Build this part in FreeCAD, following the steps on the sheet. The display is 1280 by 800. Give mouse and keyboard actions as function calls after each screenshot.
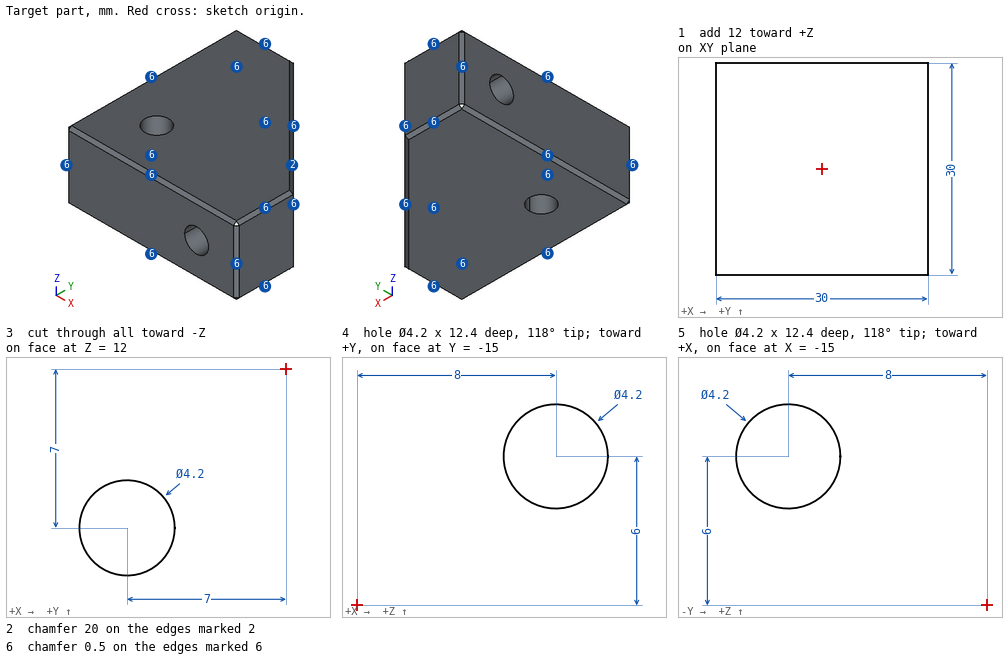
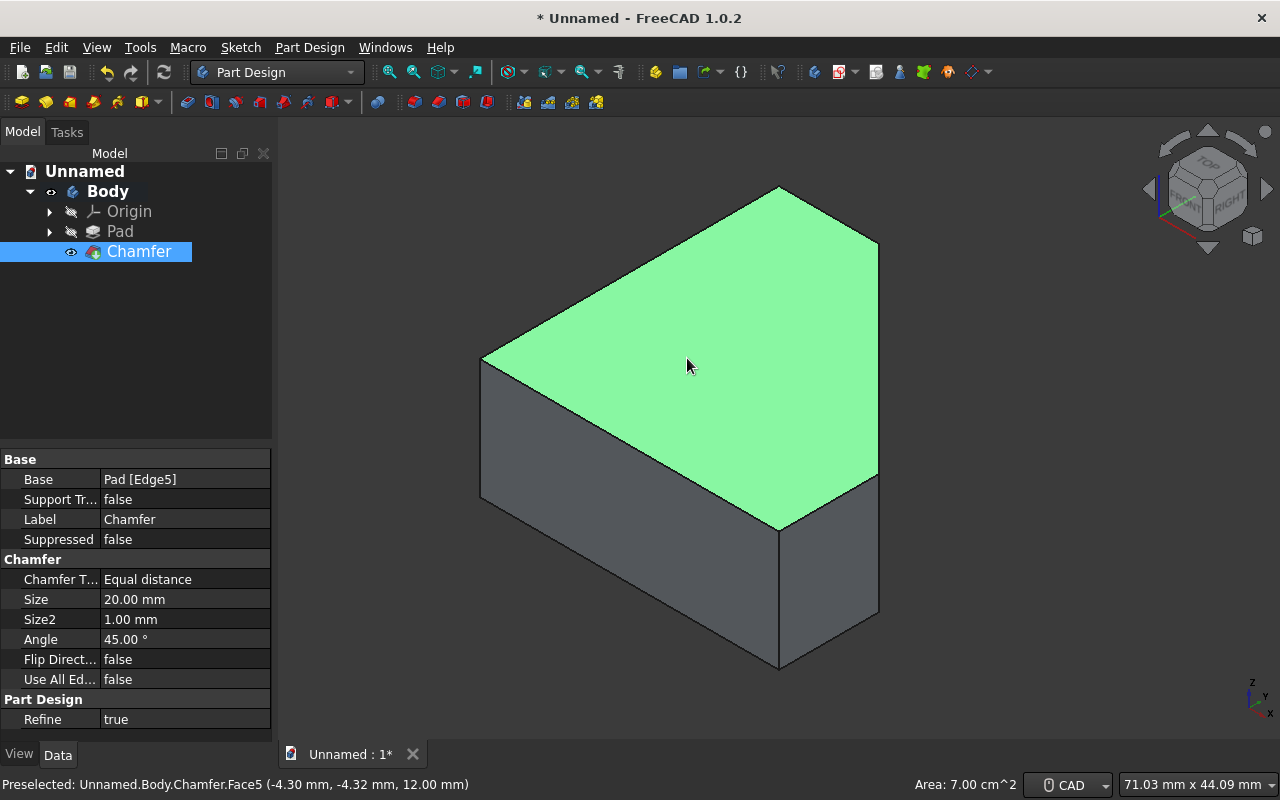
click(840, 72)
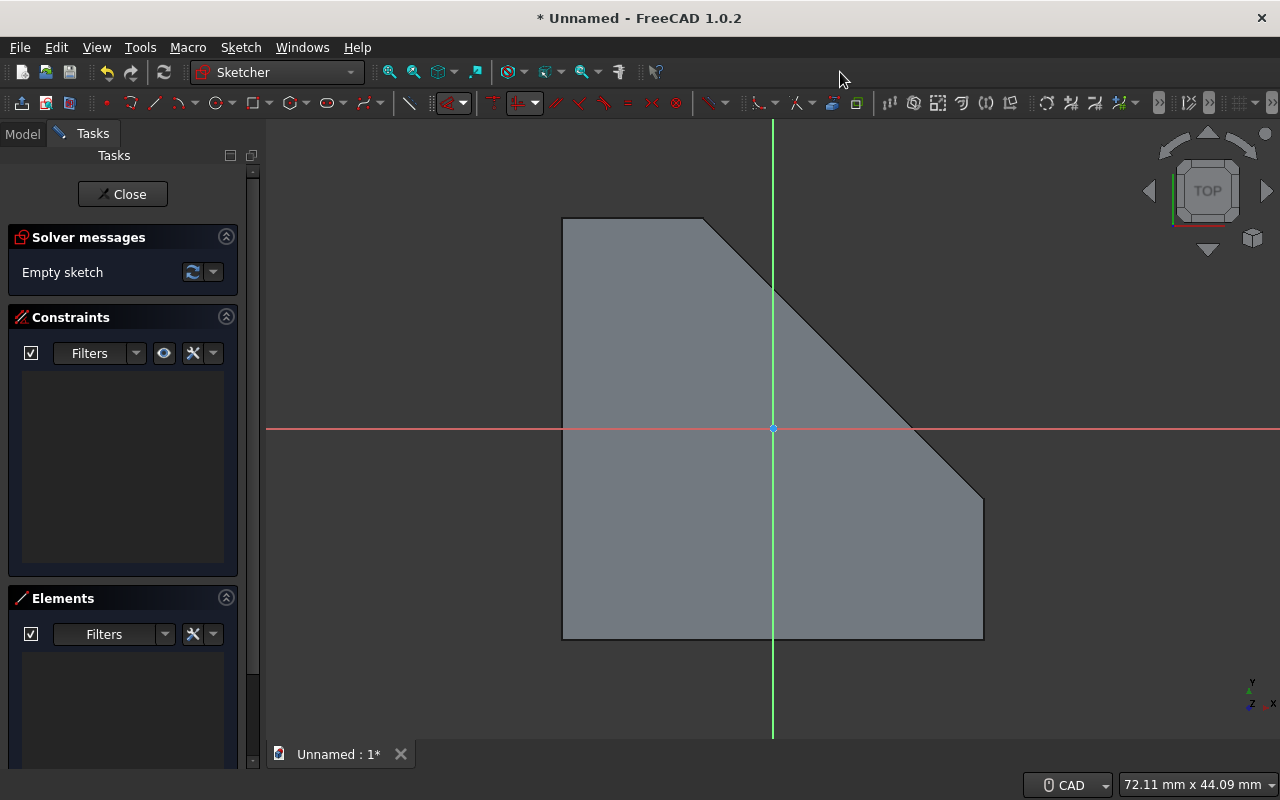
scroll(711, 521, up, 6)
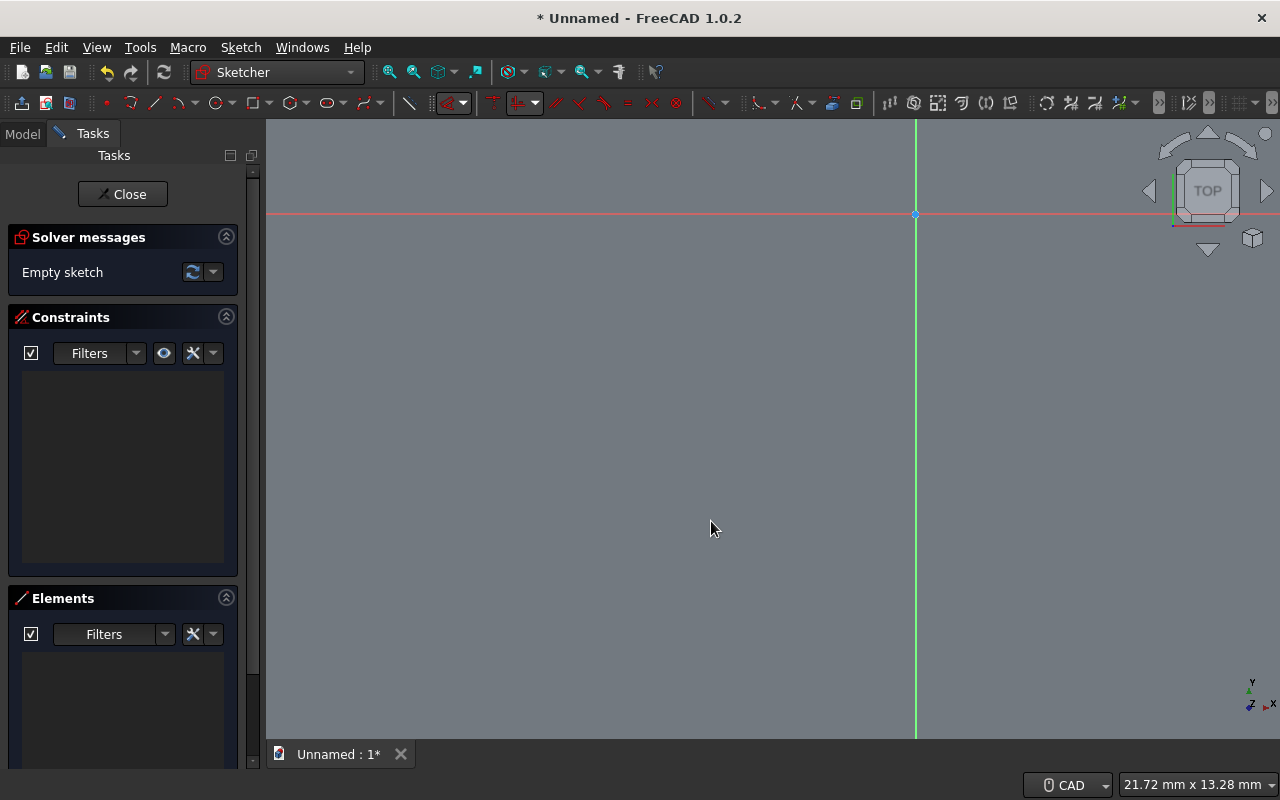
key(g)
key(c)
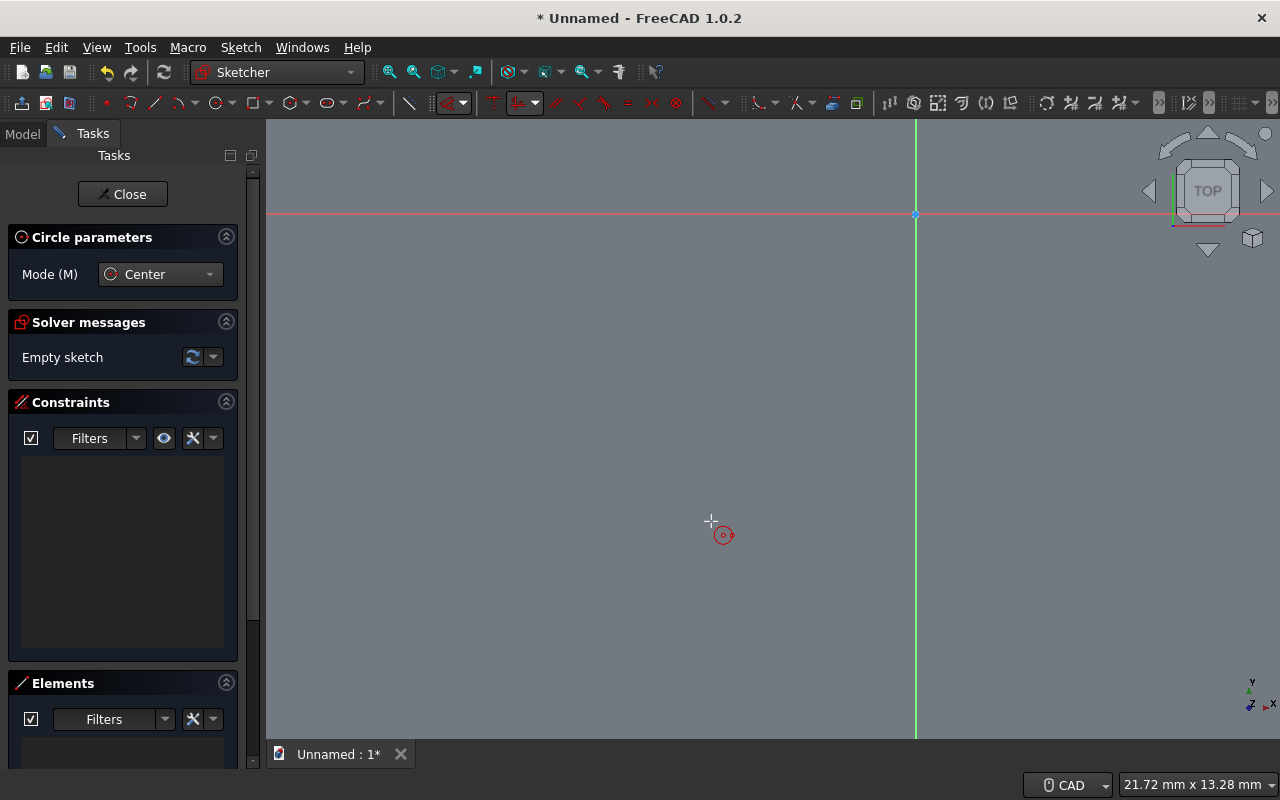
click(589, 541)
click(658, 472)
key(Escape)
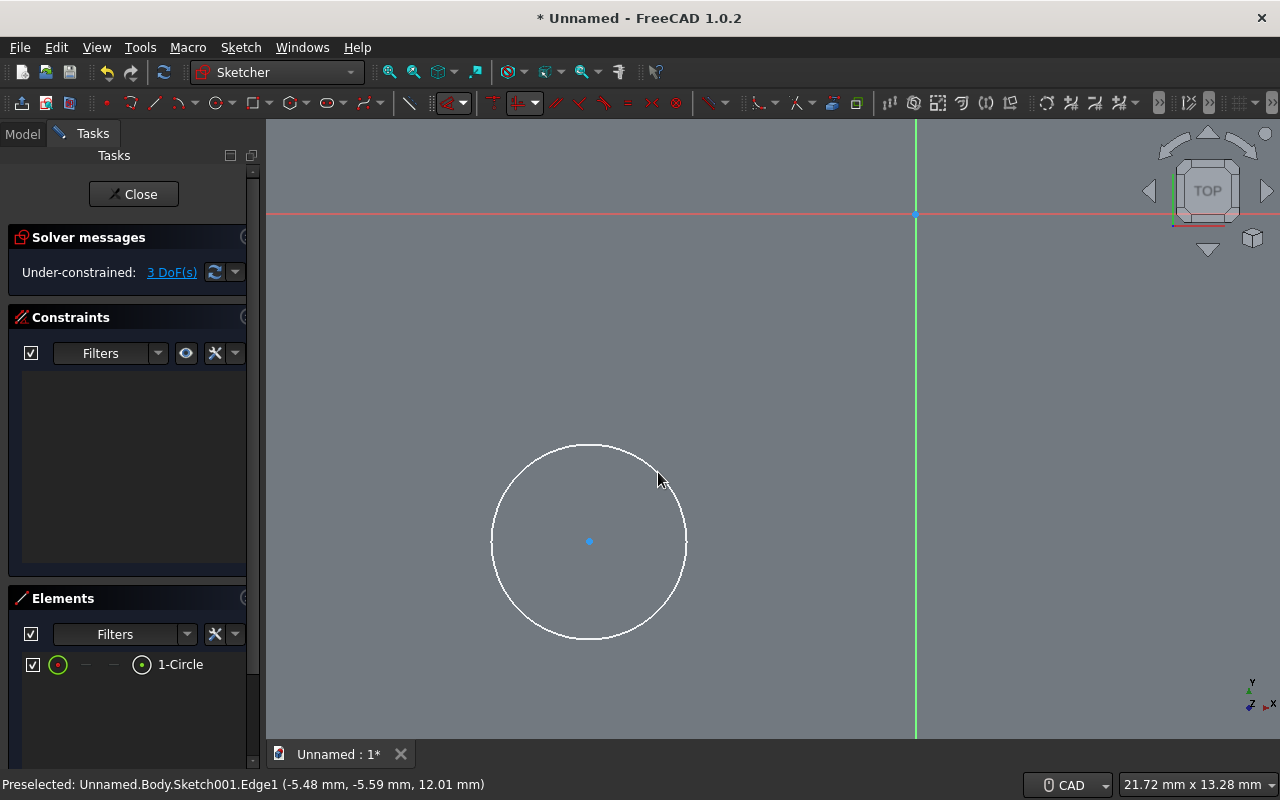
click(448, 104)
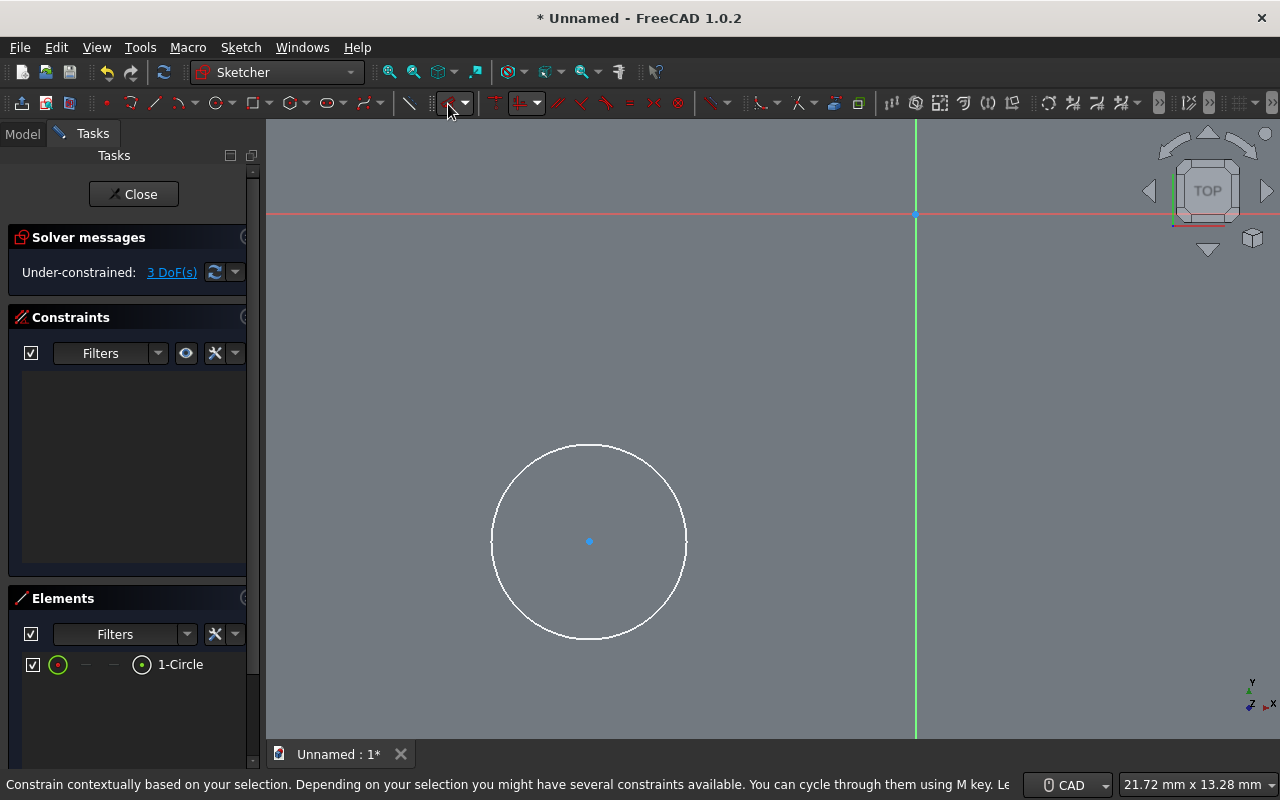
click(658, 473)
click(681, 450)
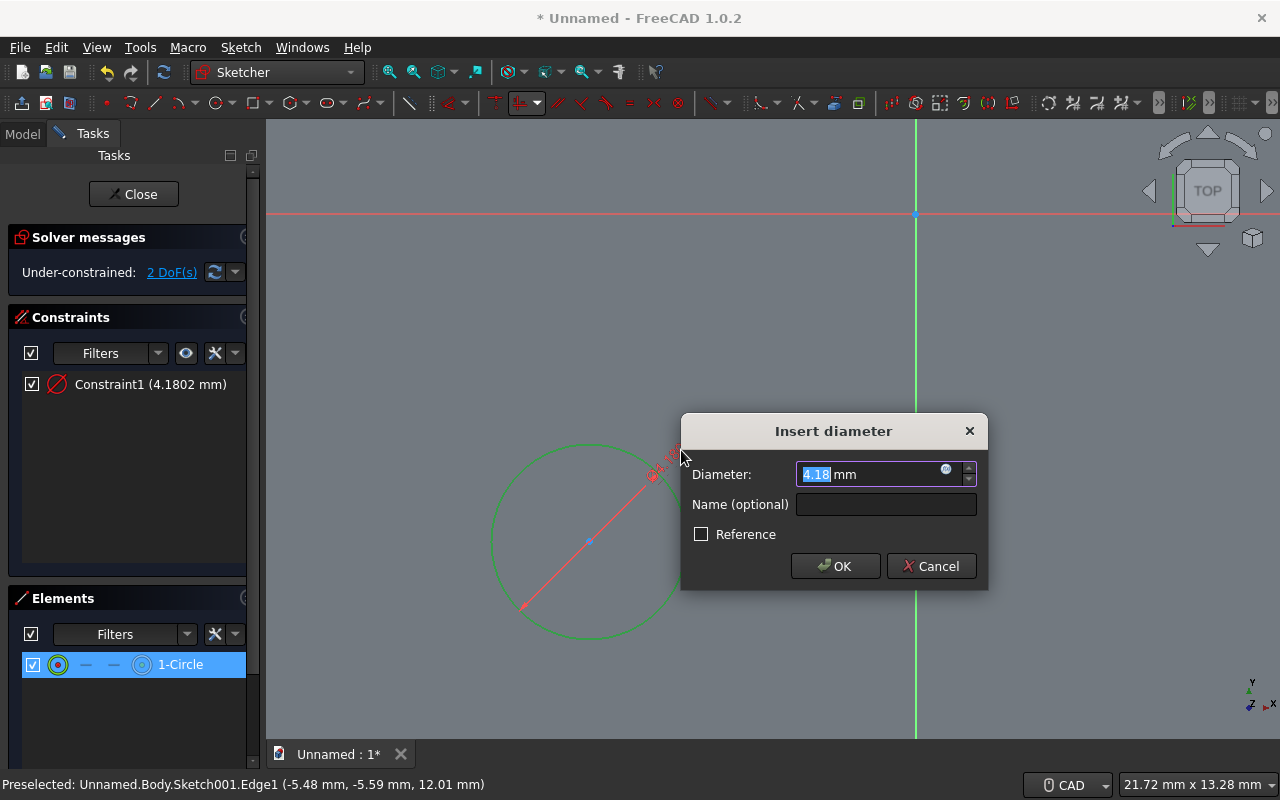
text(4.2)
key(Return)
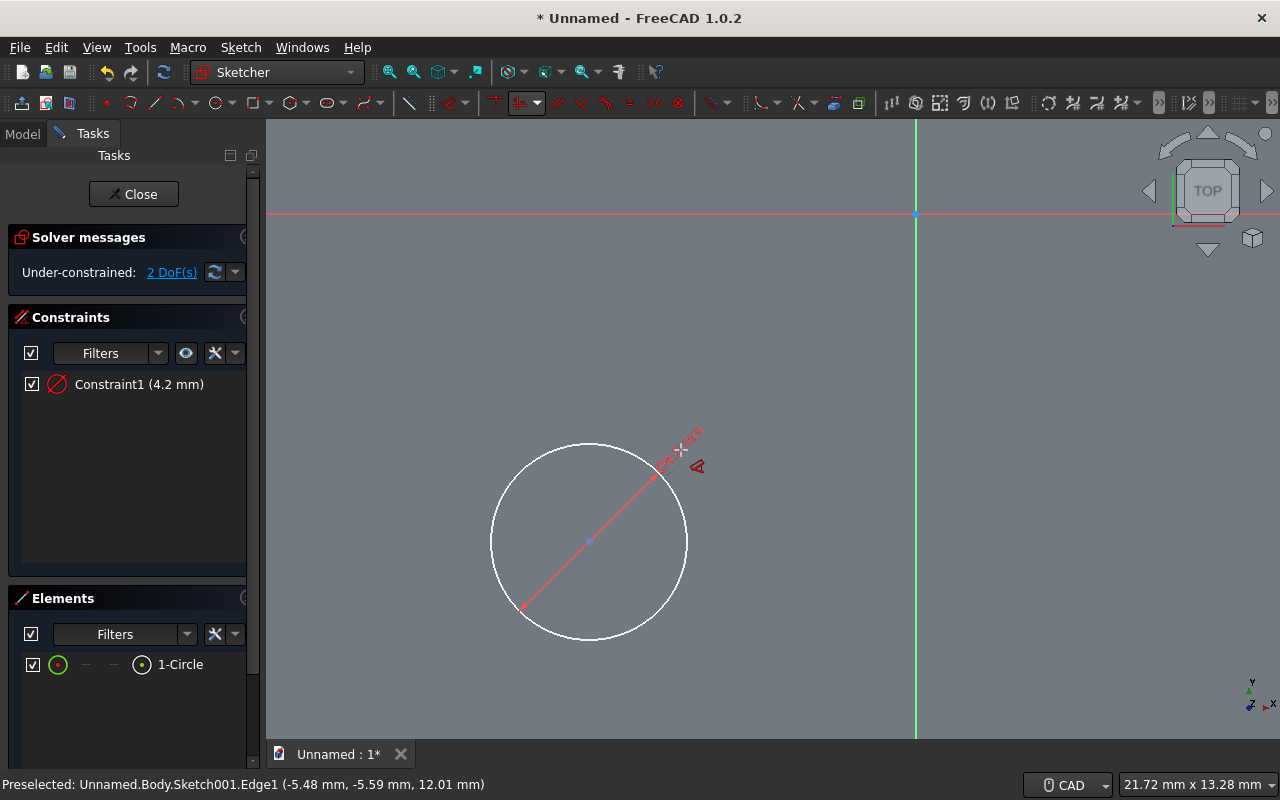
click(589, 542)
click(752, 180)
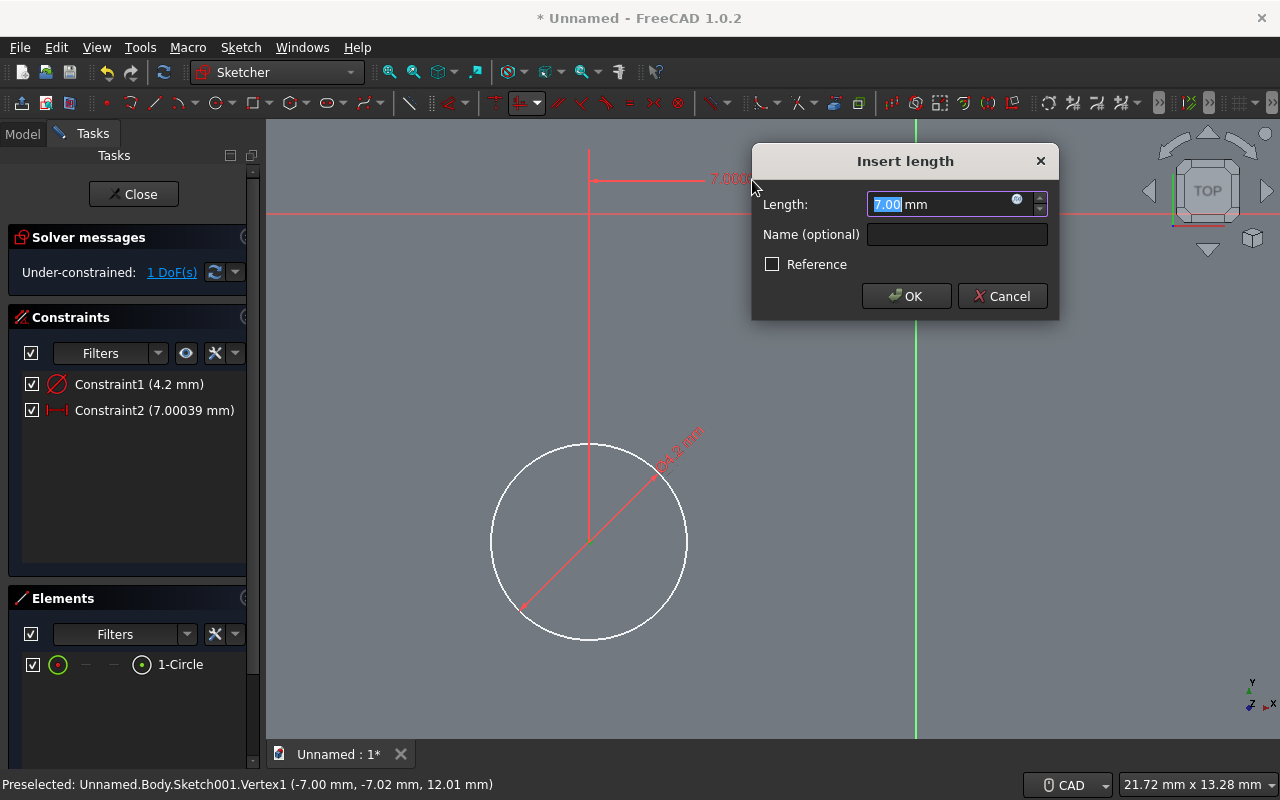
text(7)
key(Return)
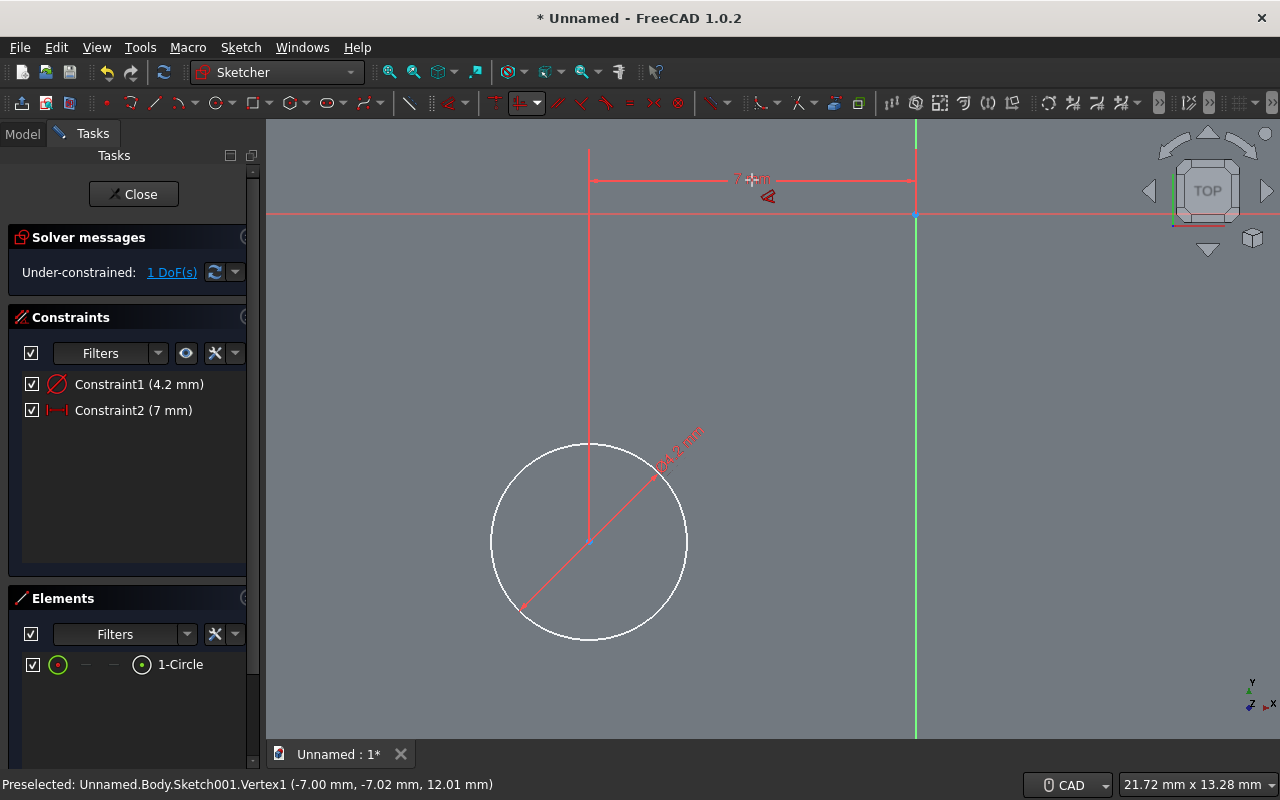
click(589, 542)
click(950, 378)